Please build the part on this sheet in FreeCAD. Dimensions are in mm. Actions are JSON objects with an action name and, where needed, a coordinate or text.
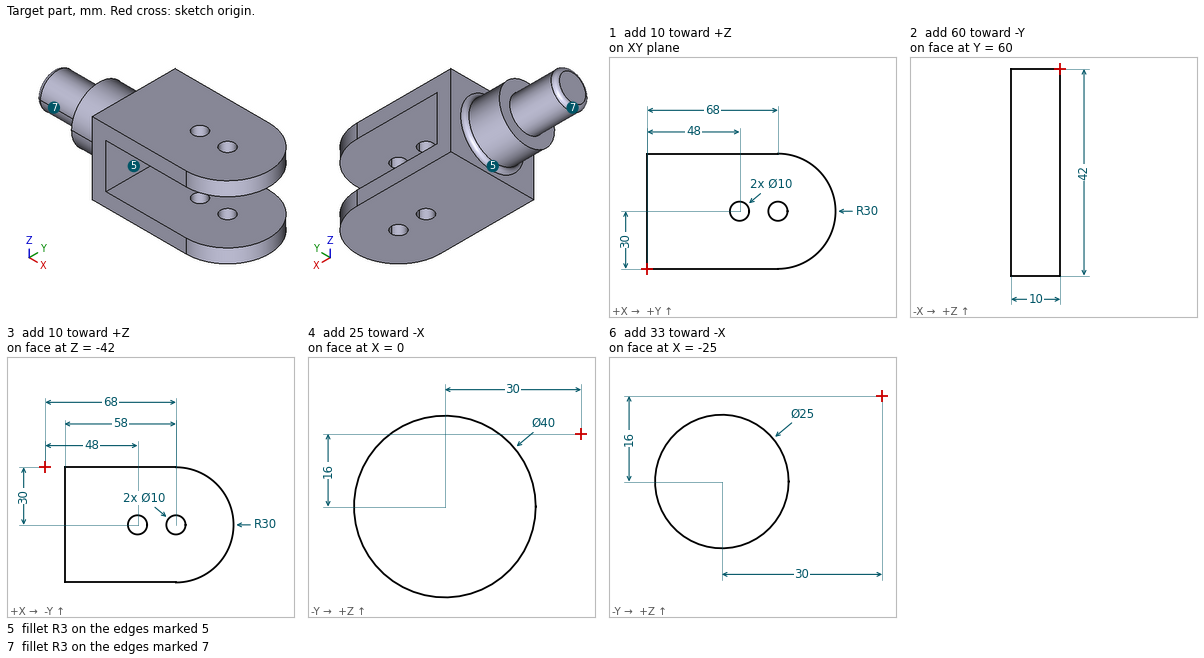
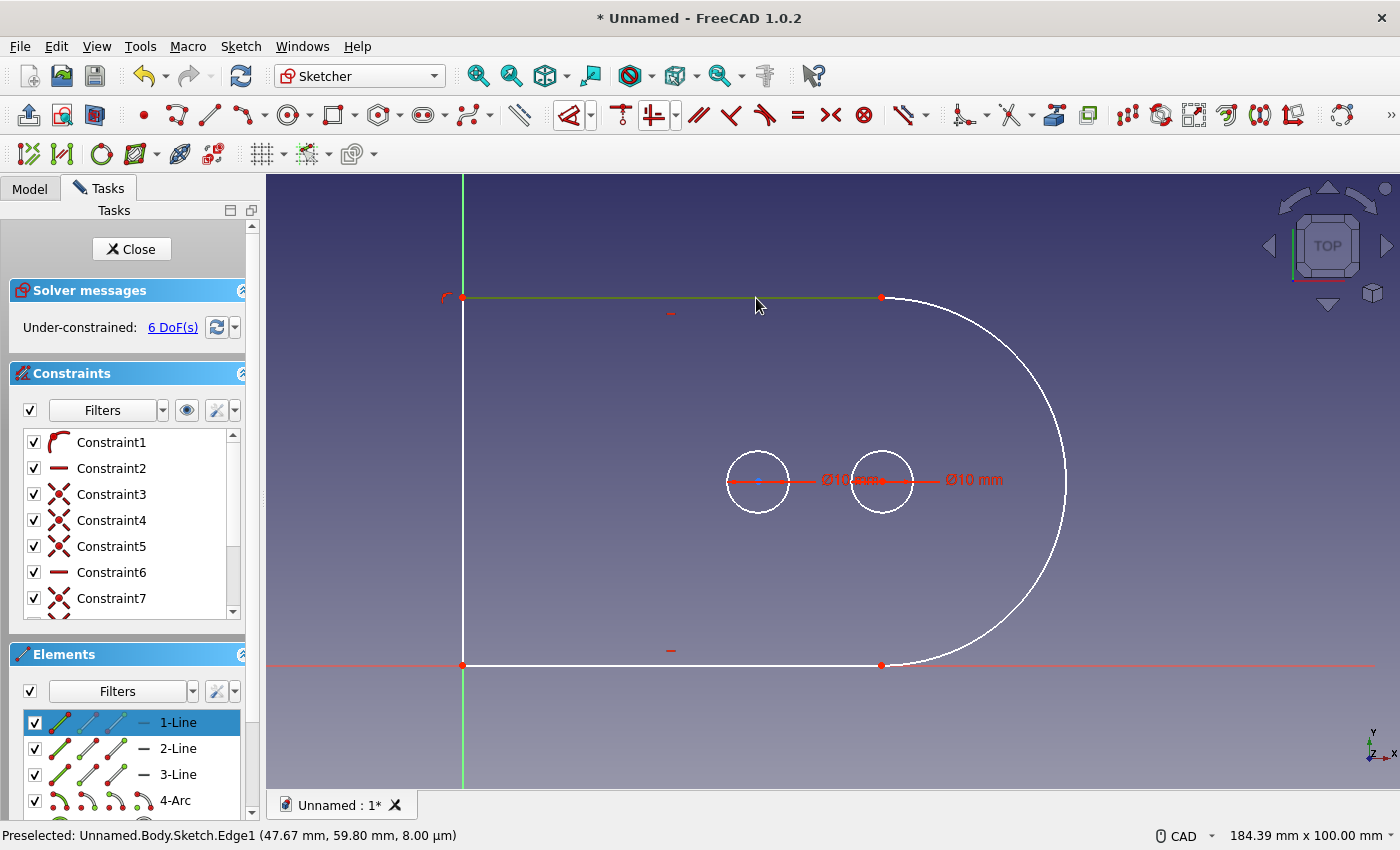
{"action": "left_click", "coordinate": [1031, 590]}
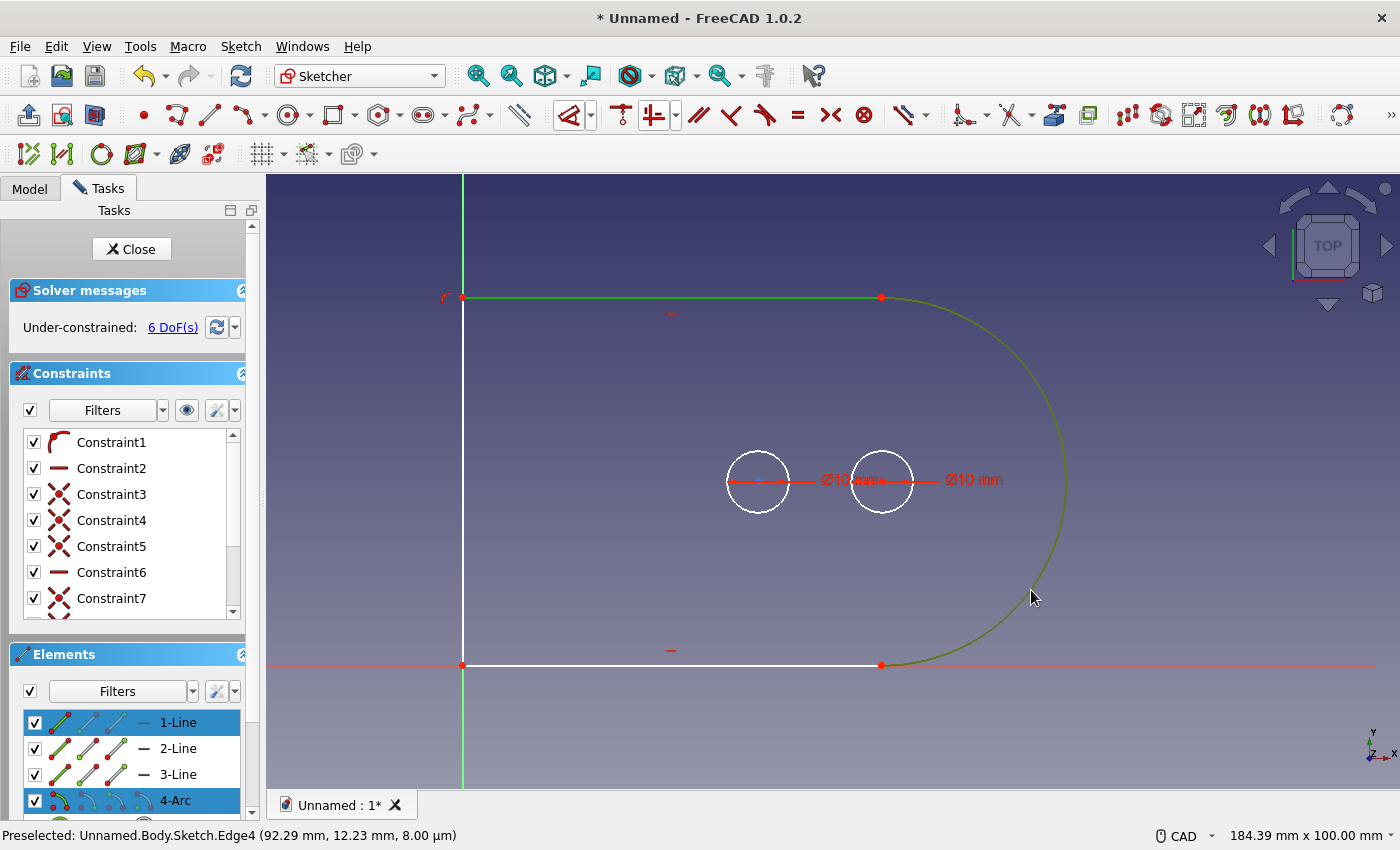
{"action": "key", "text": "t"}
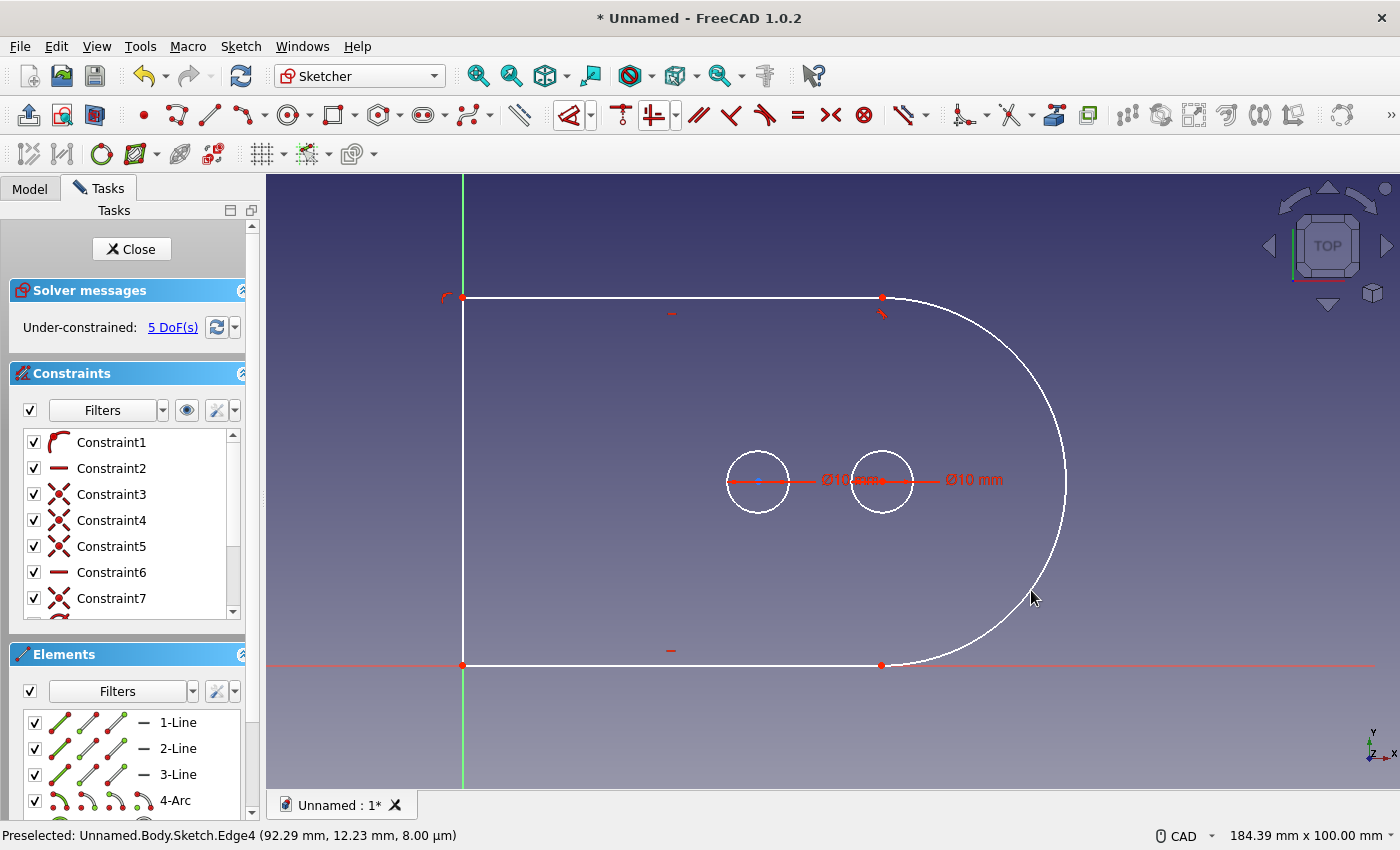
{"action": "left_click", "coordinate": [588, 666]}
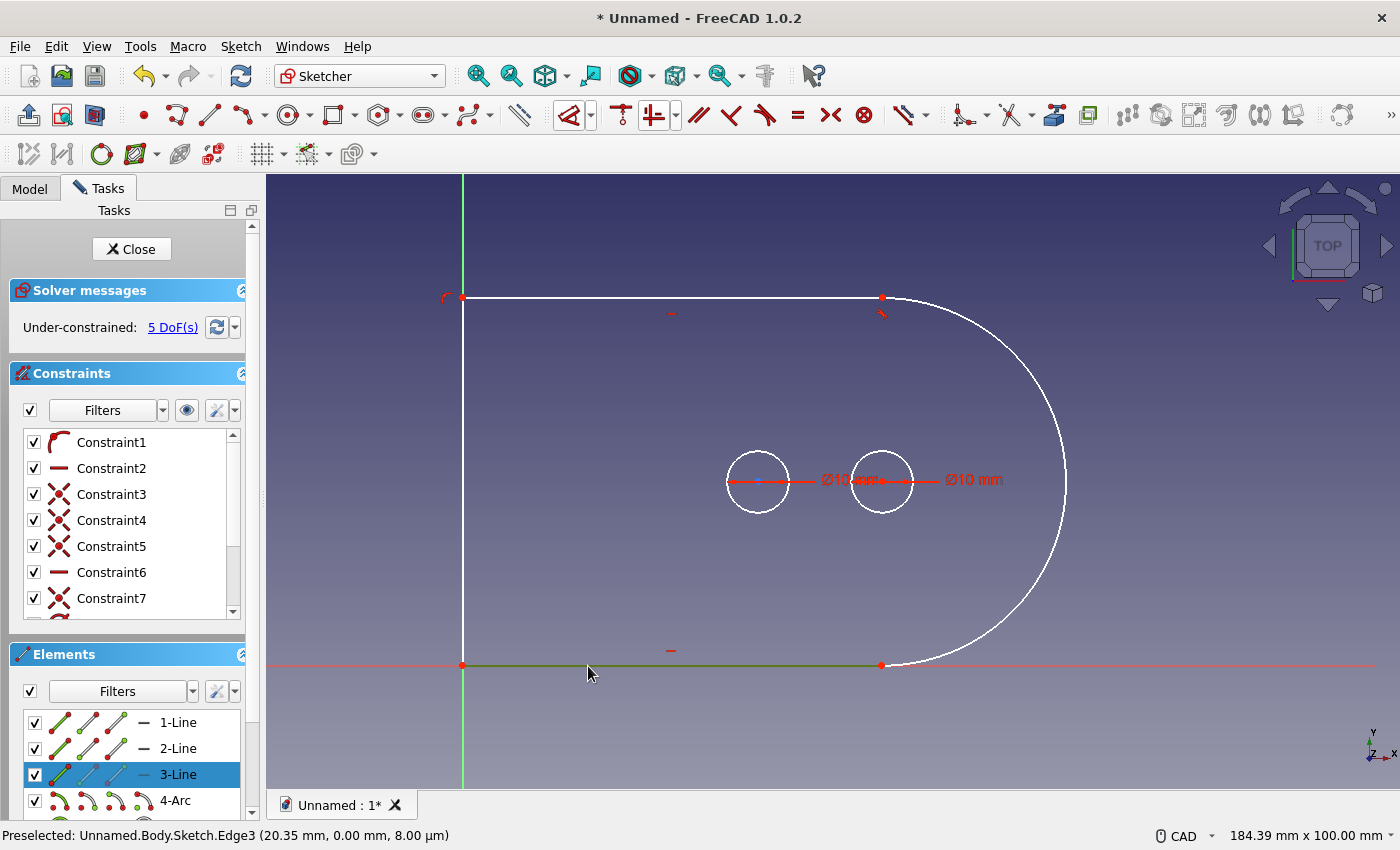
{"action": "left_click", "coordinate": [1030, 591]}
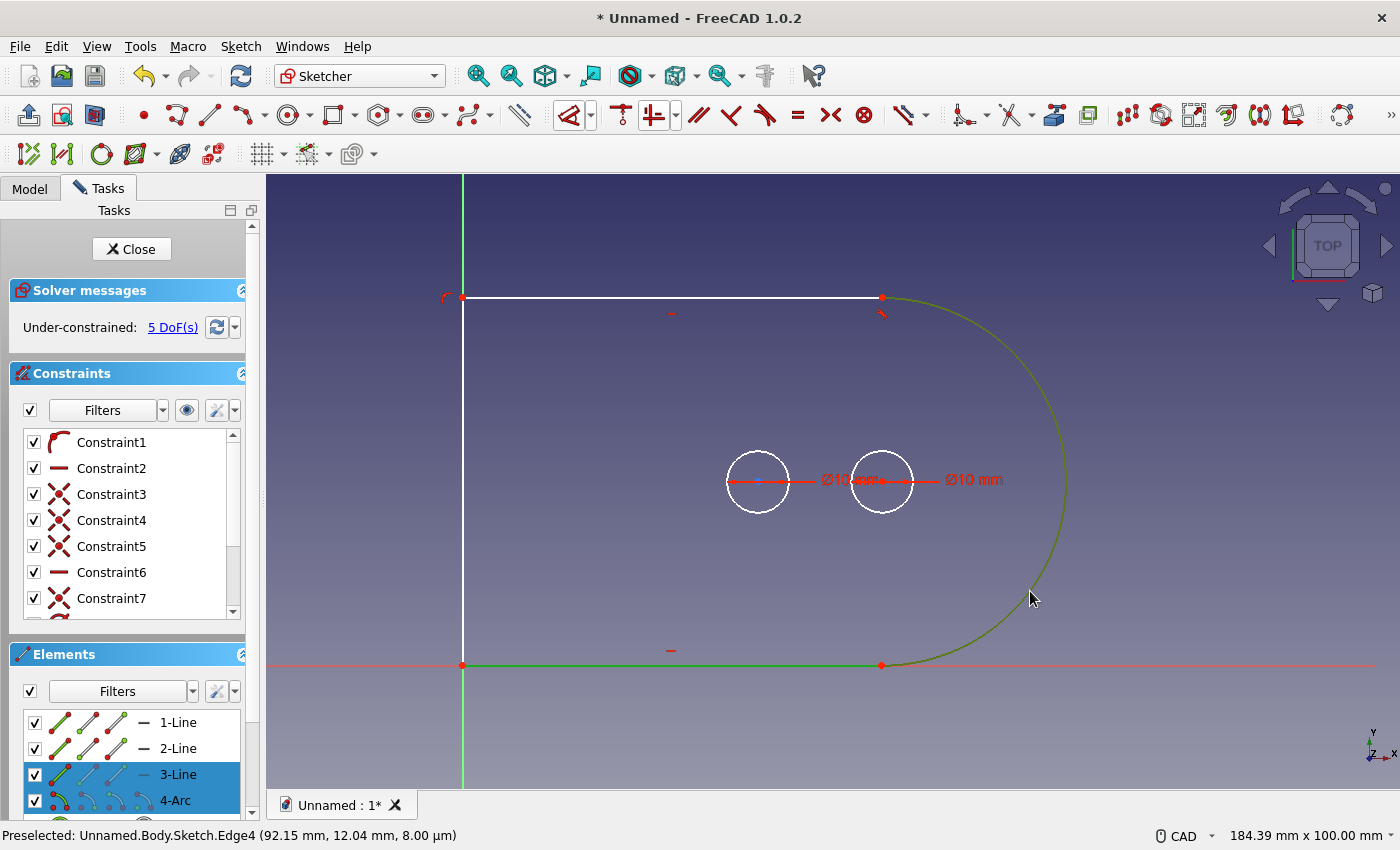
{"action": "key", "text": "t"}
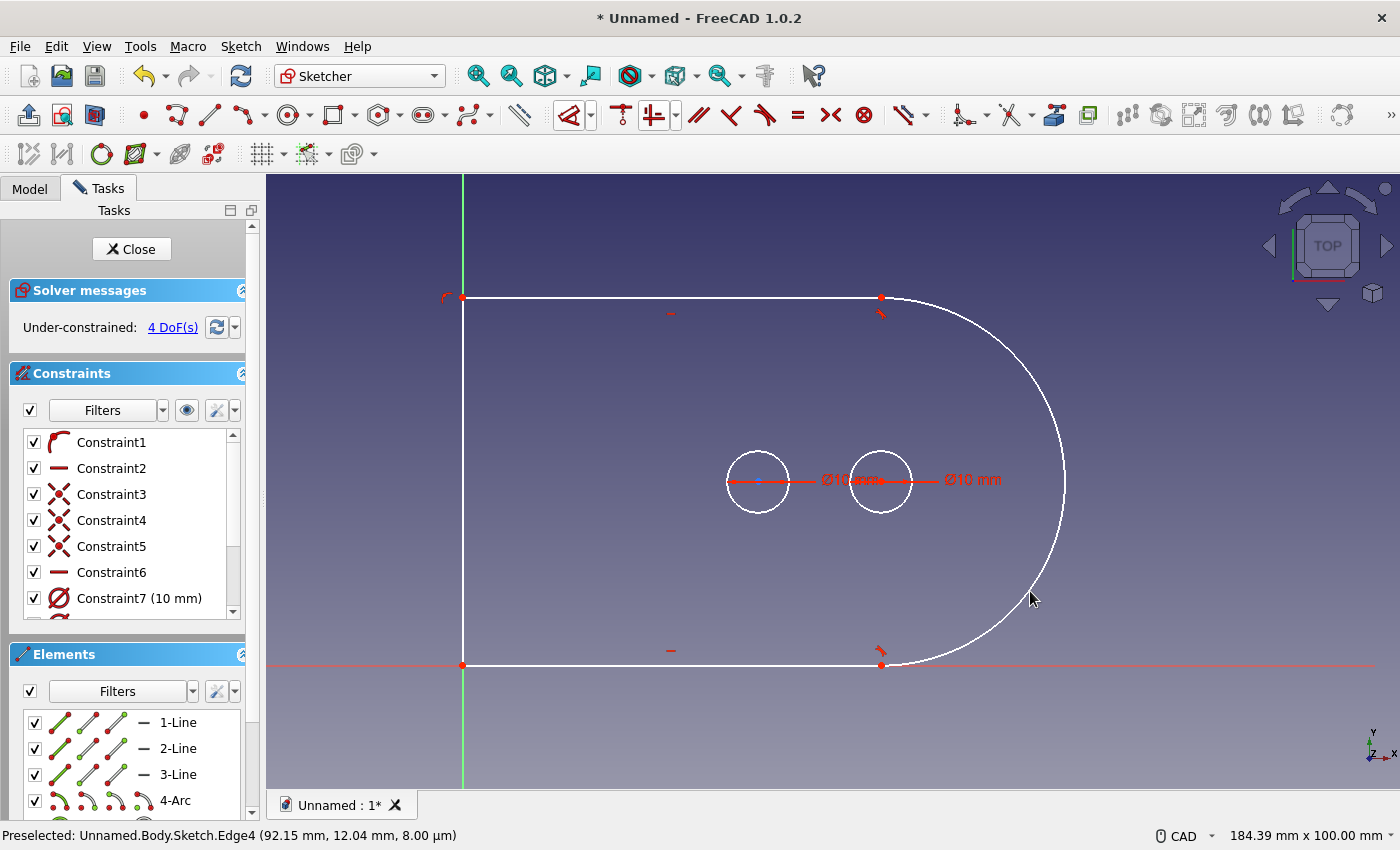
{"action": "key", "text": "d"}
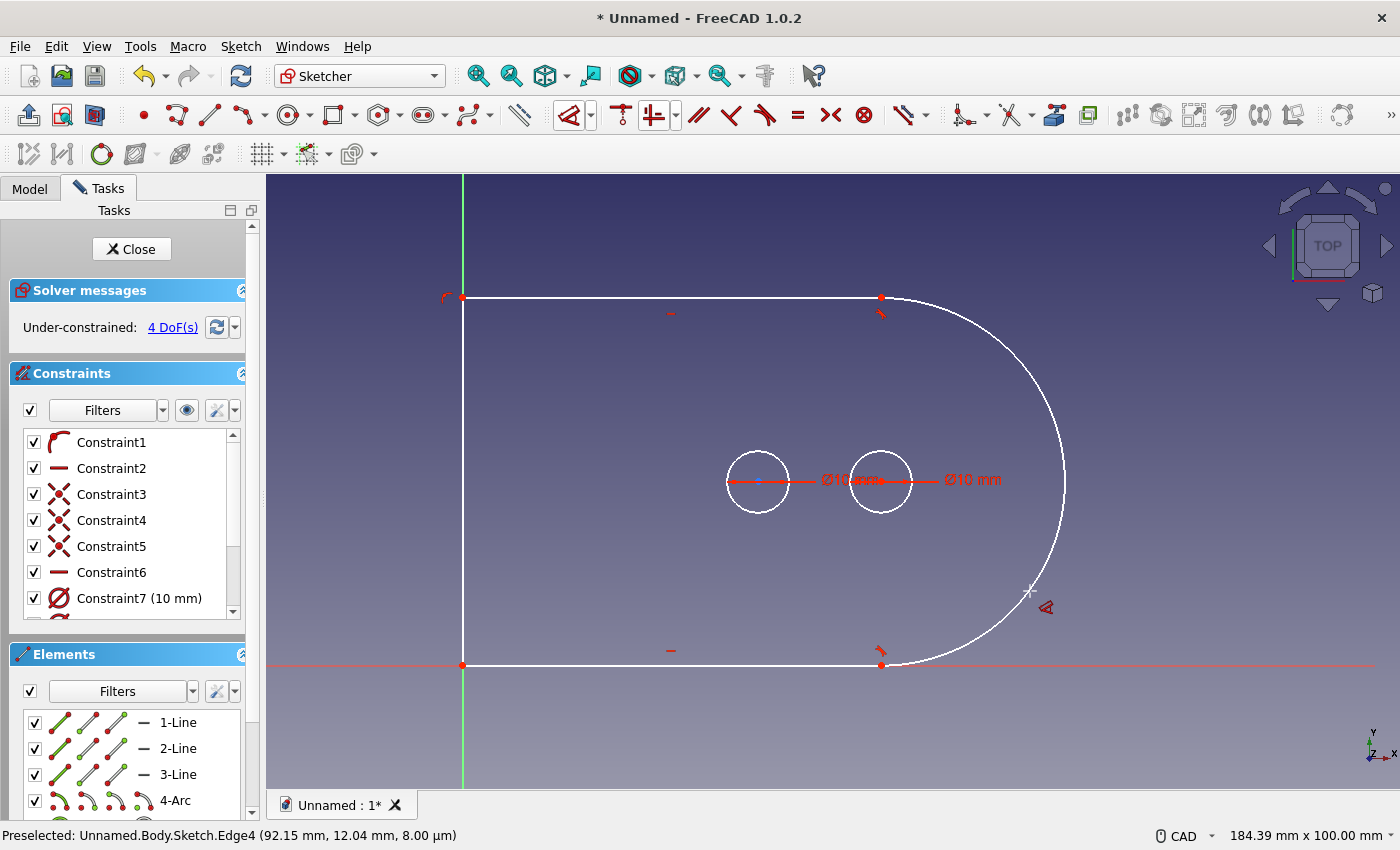
{"action": "left_click", "coordinate": [1030, 590]}
{"action": "left_click", "coordinate": [1056, 609]}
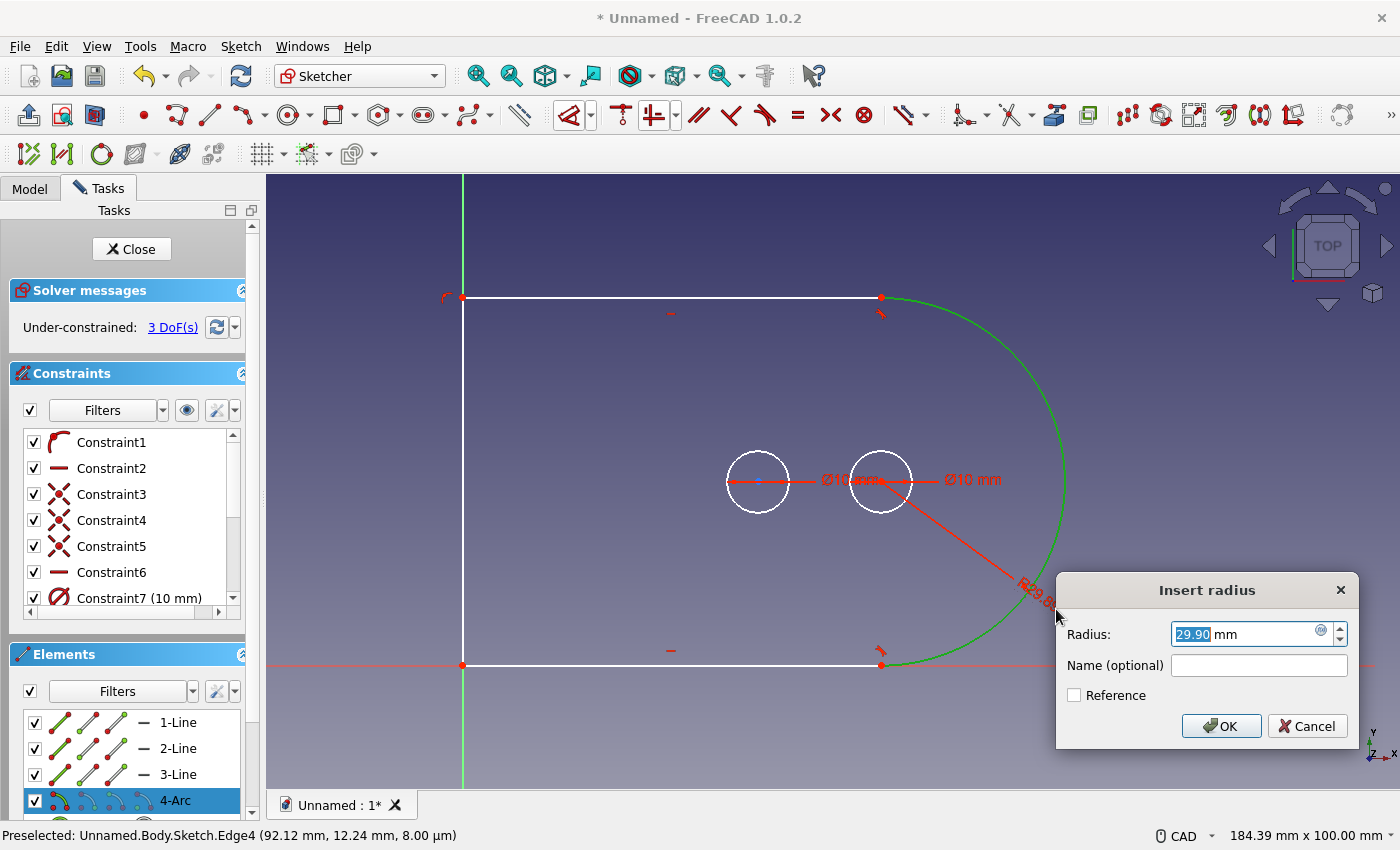
{"action": "type", "text": "30"}
{"action": "key", "text": "Return"}